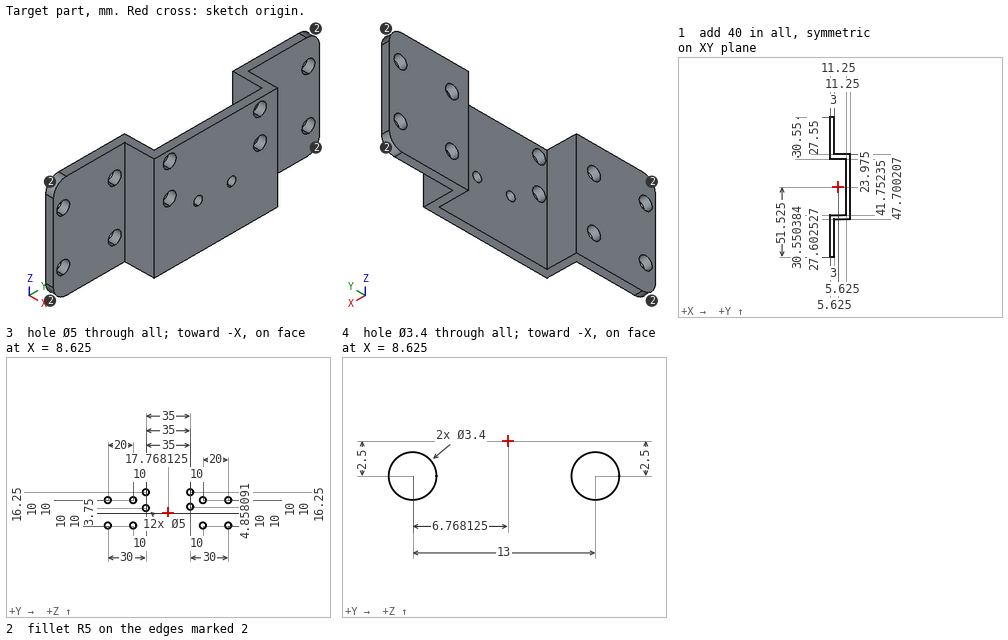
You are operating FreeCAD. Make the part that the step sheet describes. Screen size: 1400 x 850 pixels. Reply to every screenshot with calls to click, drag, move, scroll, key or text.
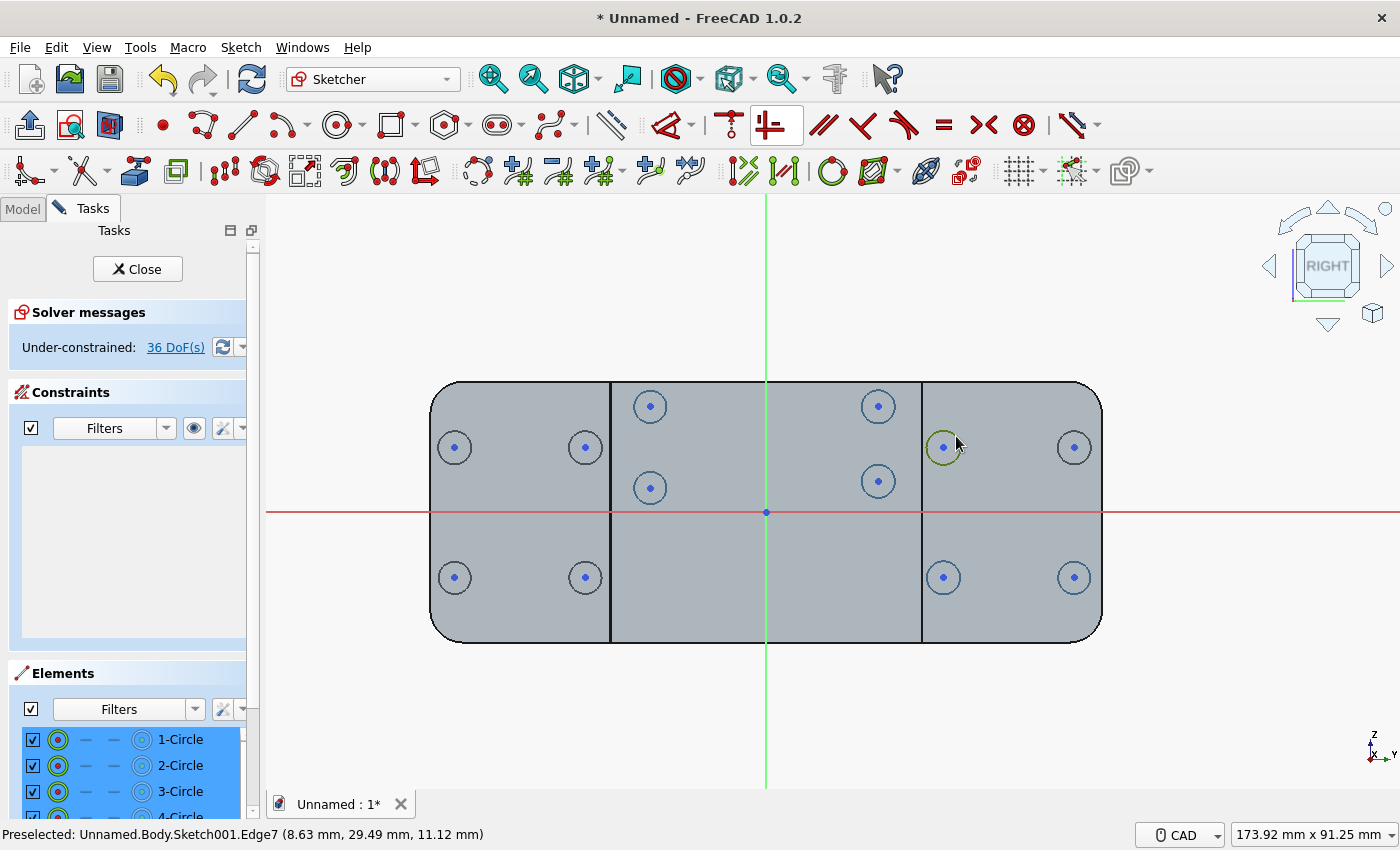
click(1086, 436)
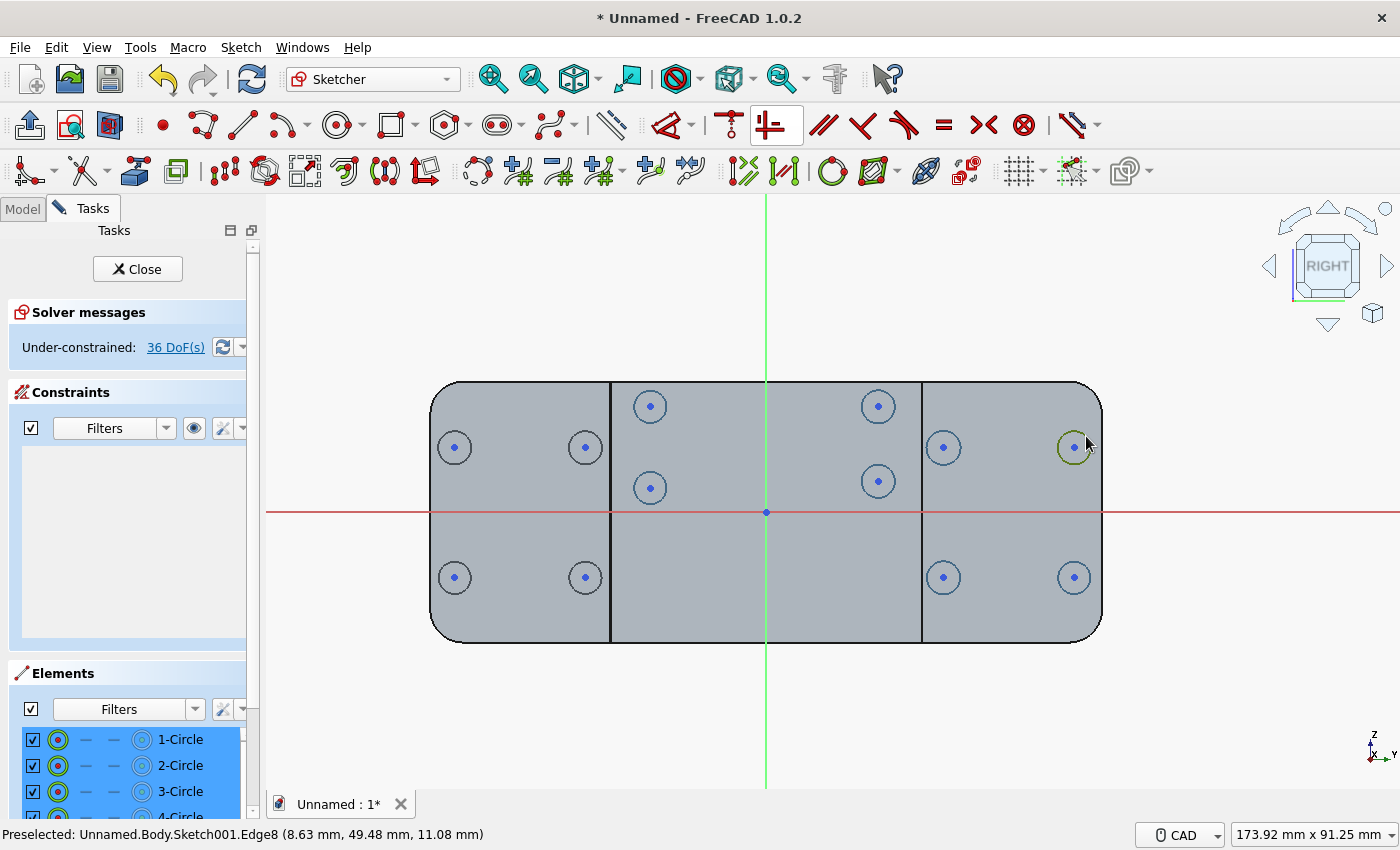
click(466, 566)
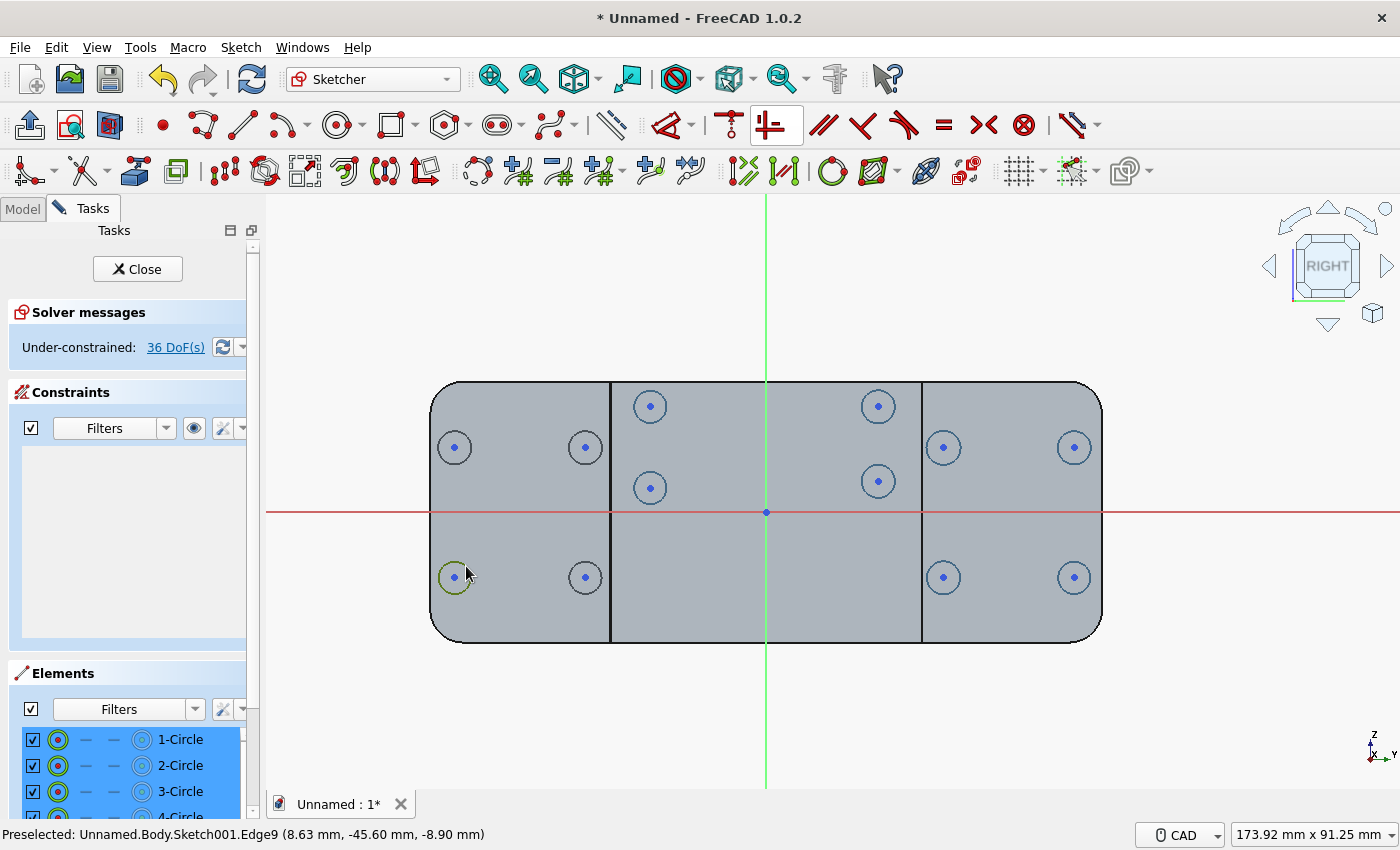
click(597, 566)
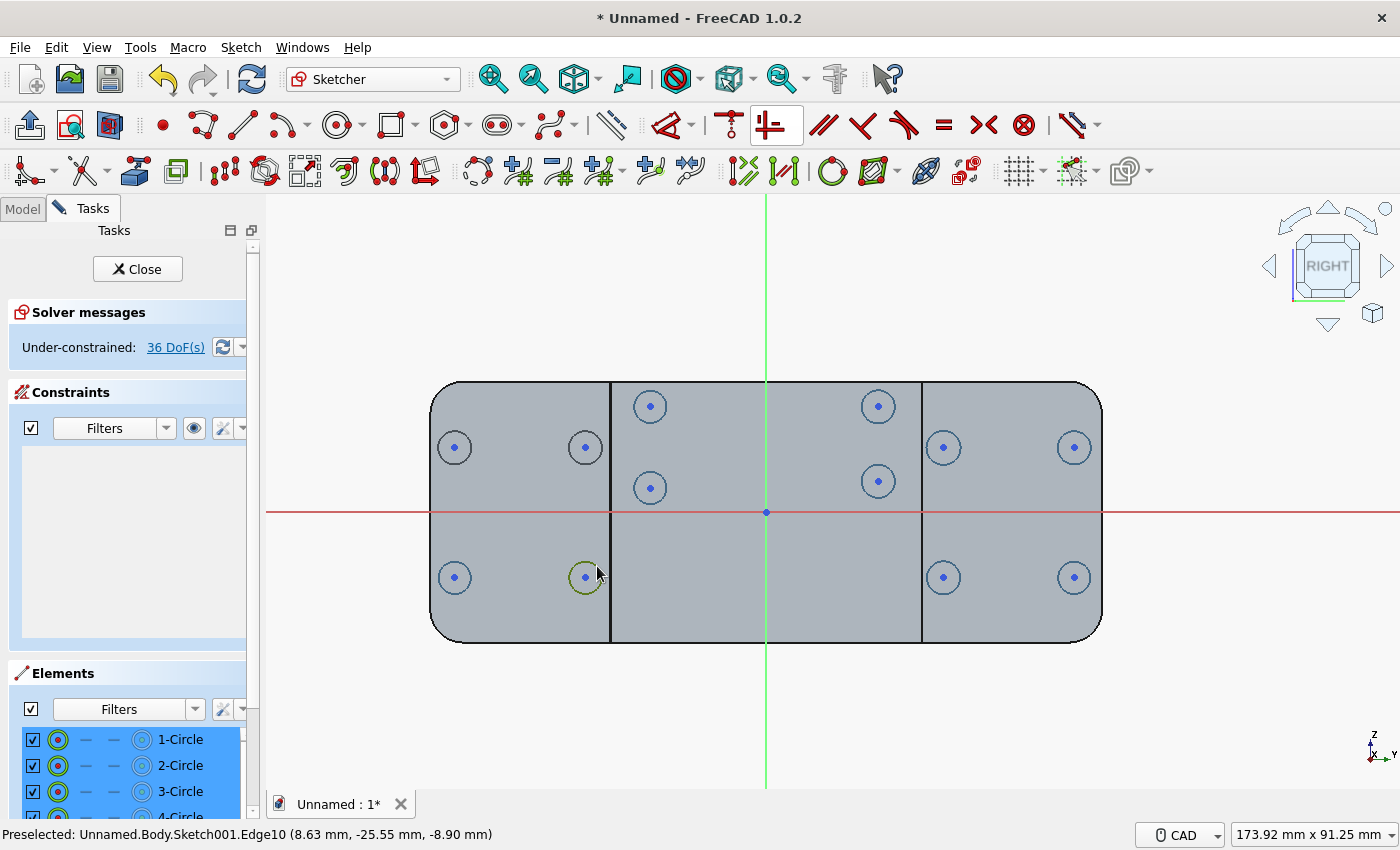
click(597, 436)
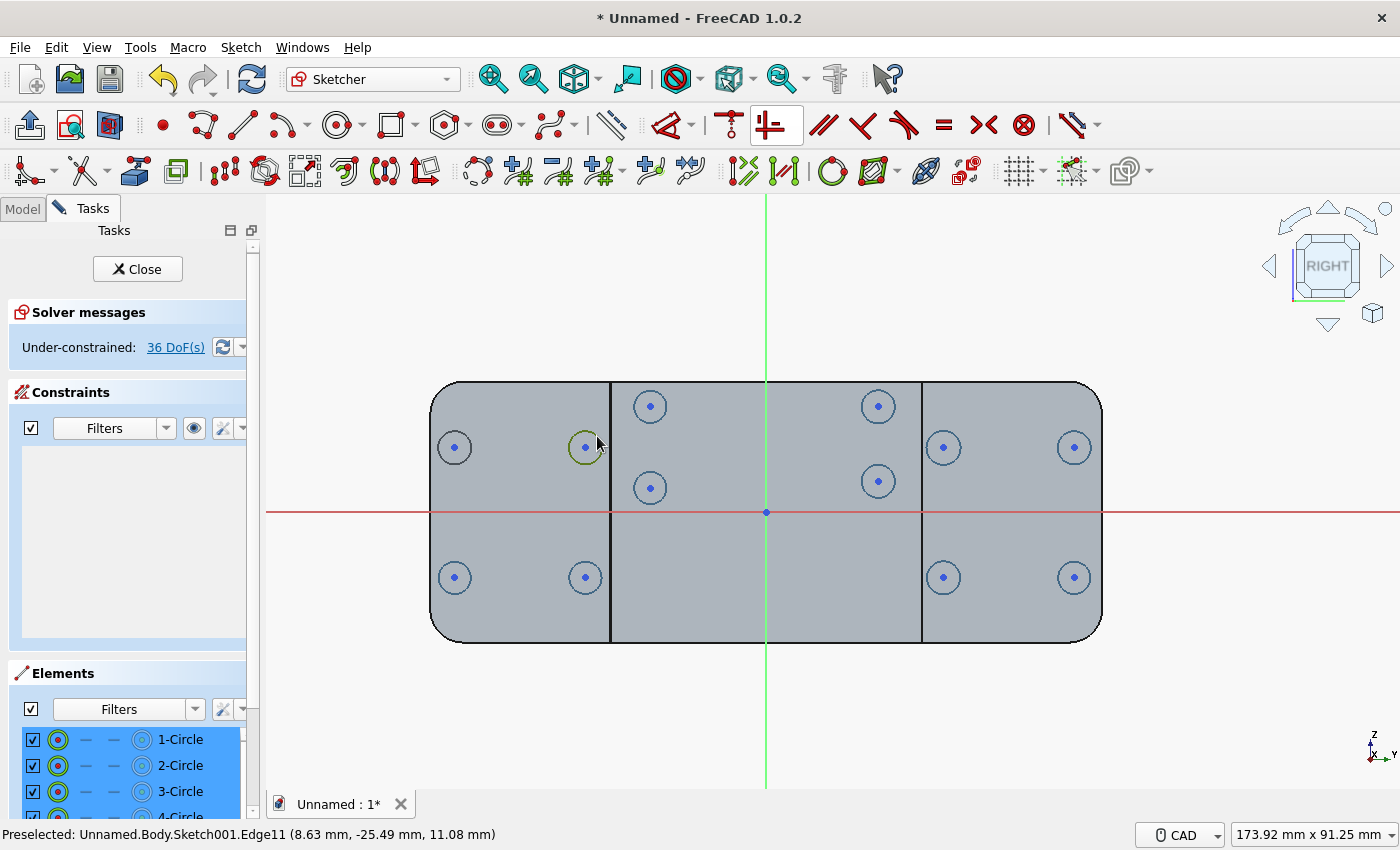
click(466, 436)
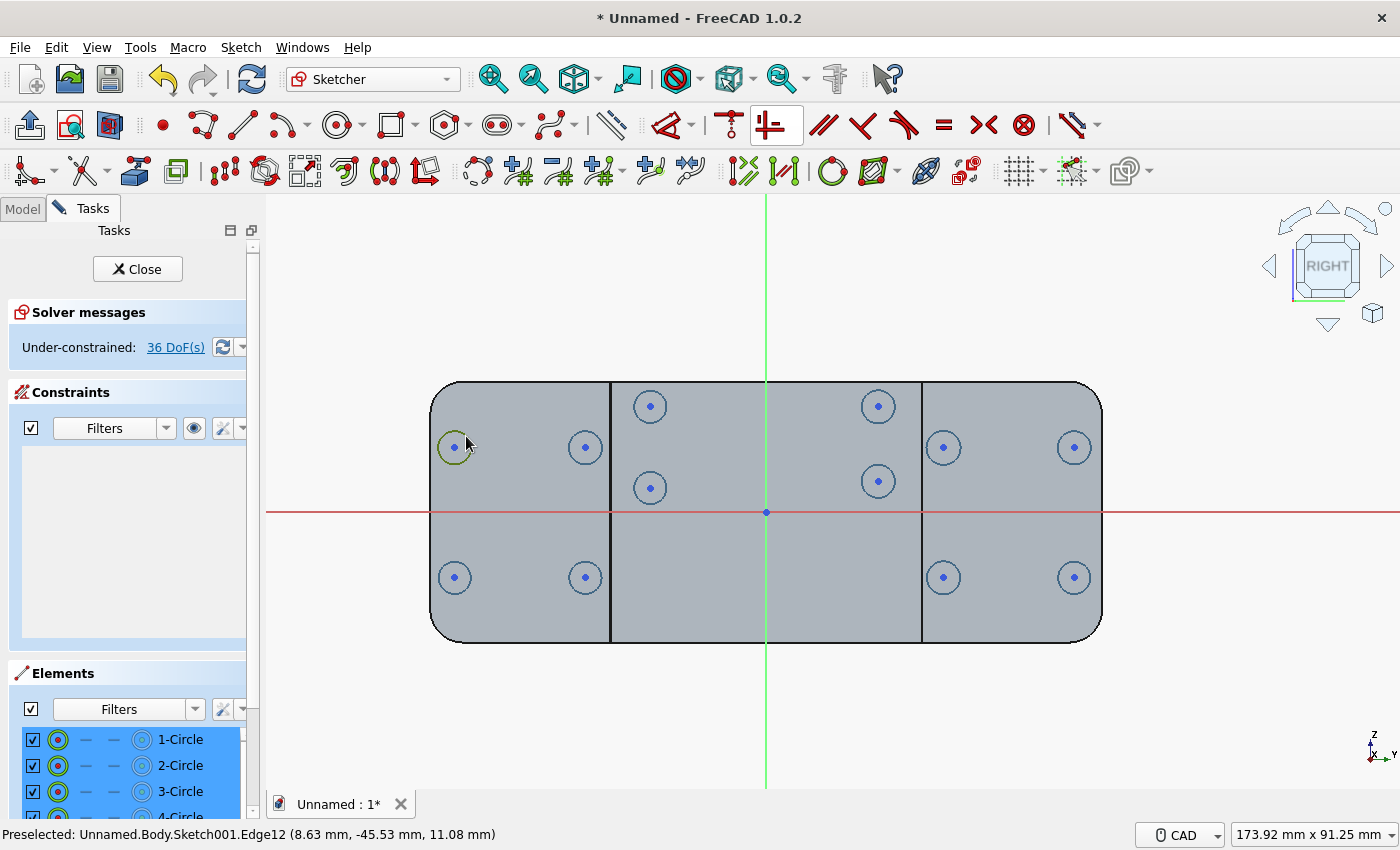
key(e)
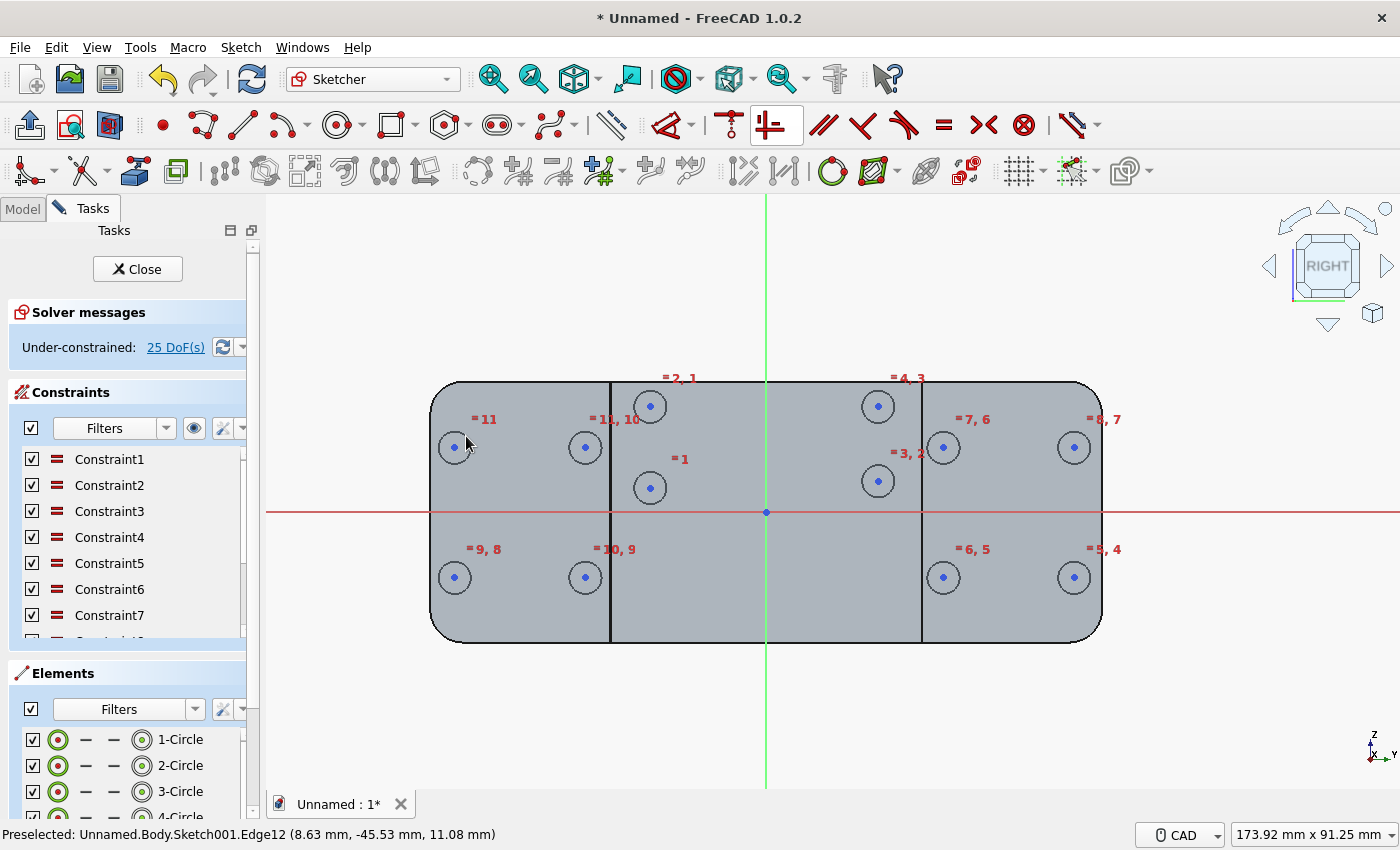
click(666, 126)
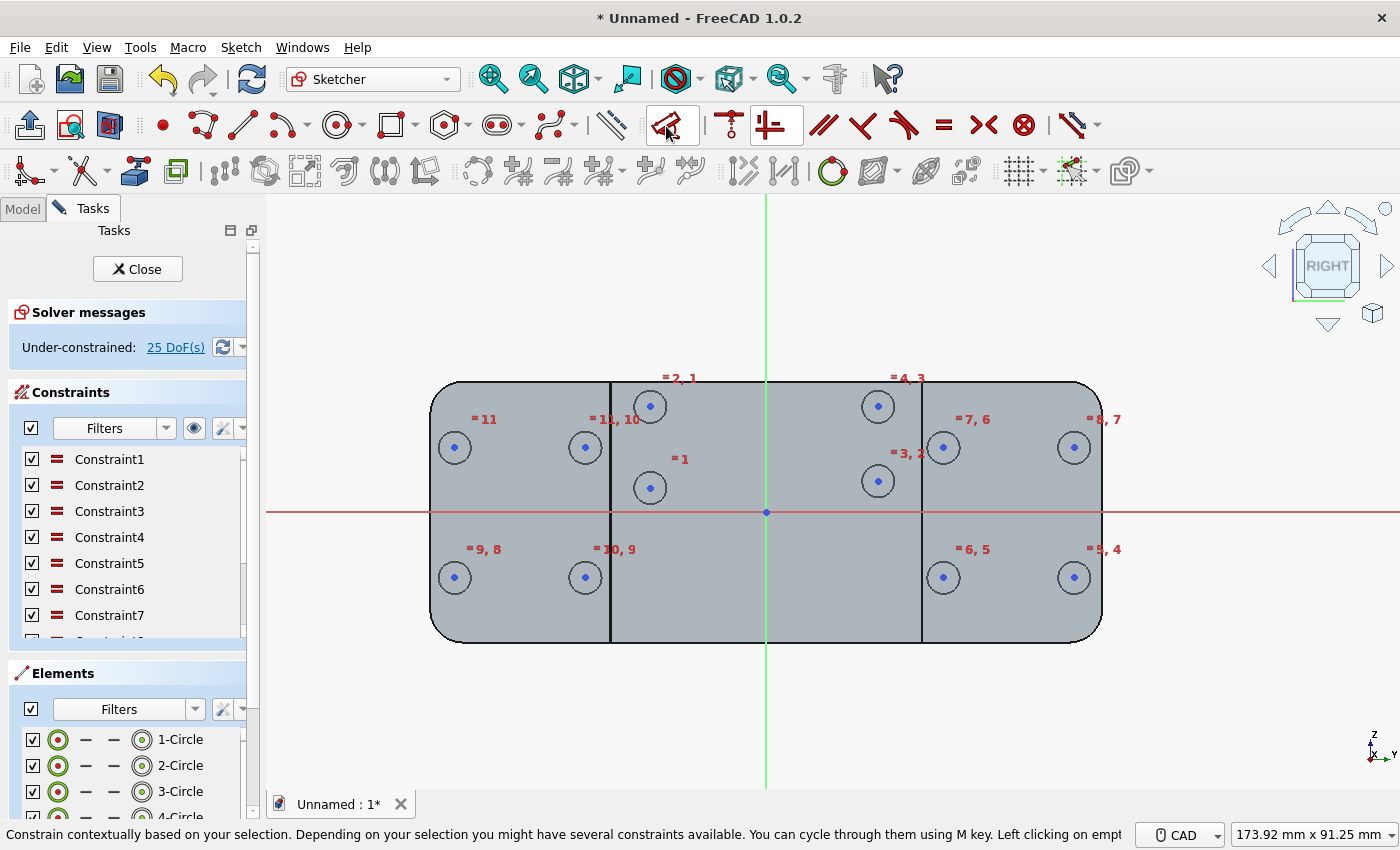
click(662, 477)
click(685, 455)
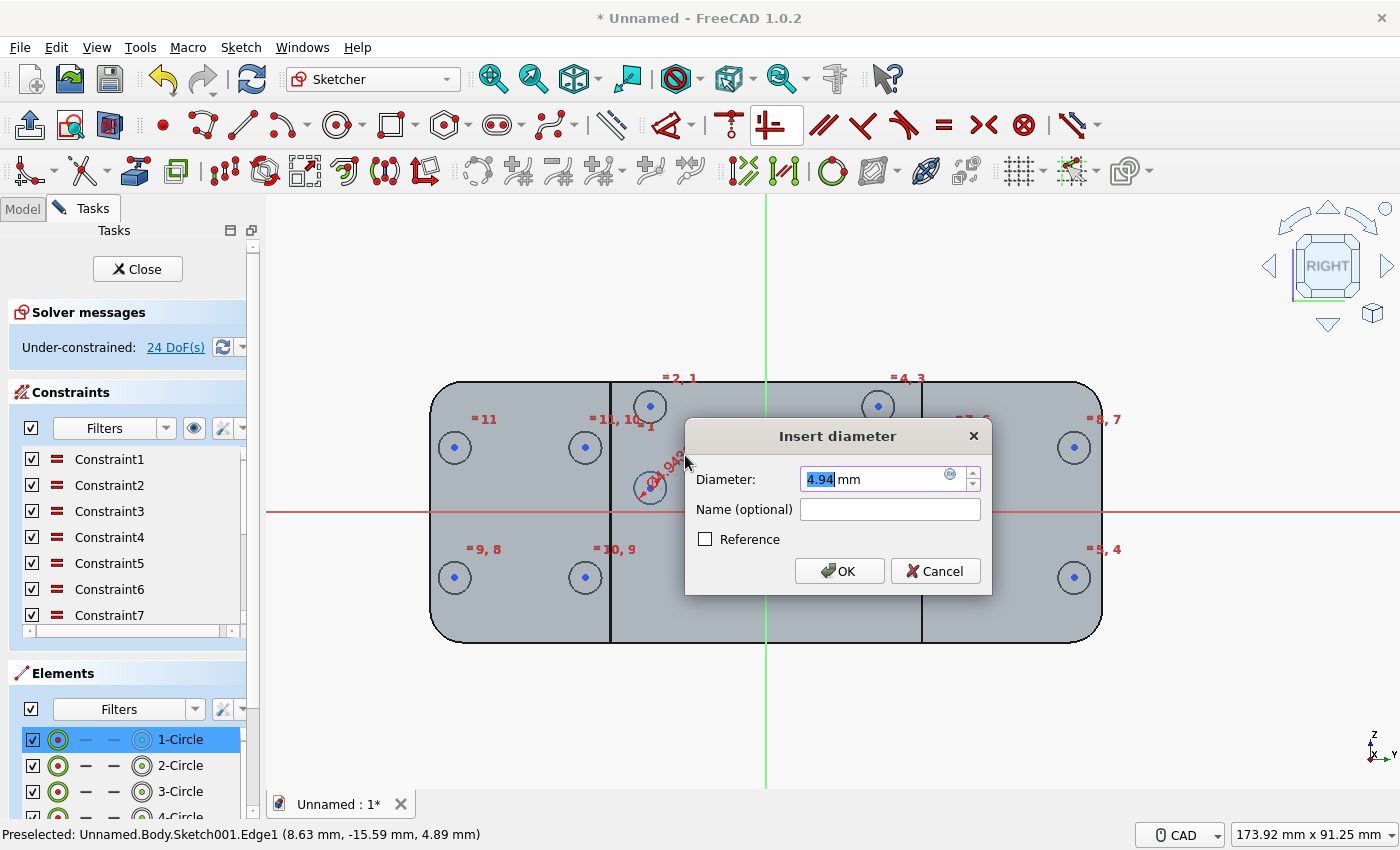
text(5)
key(Return)